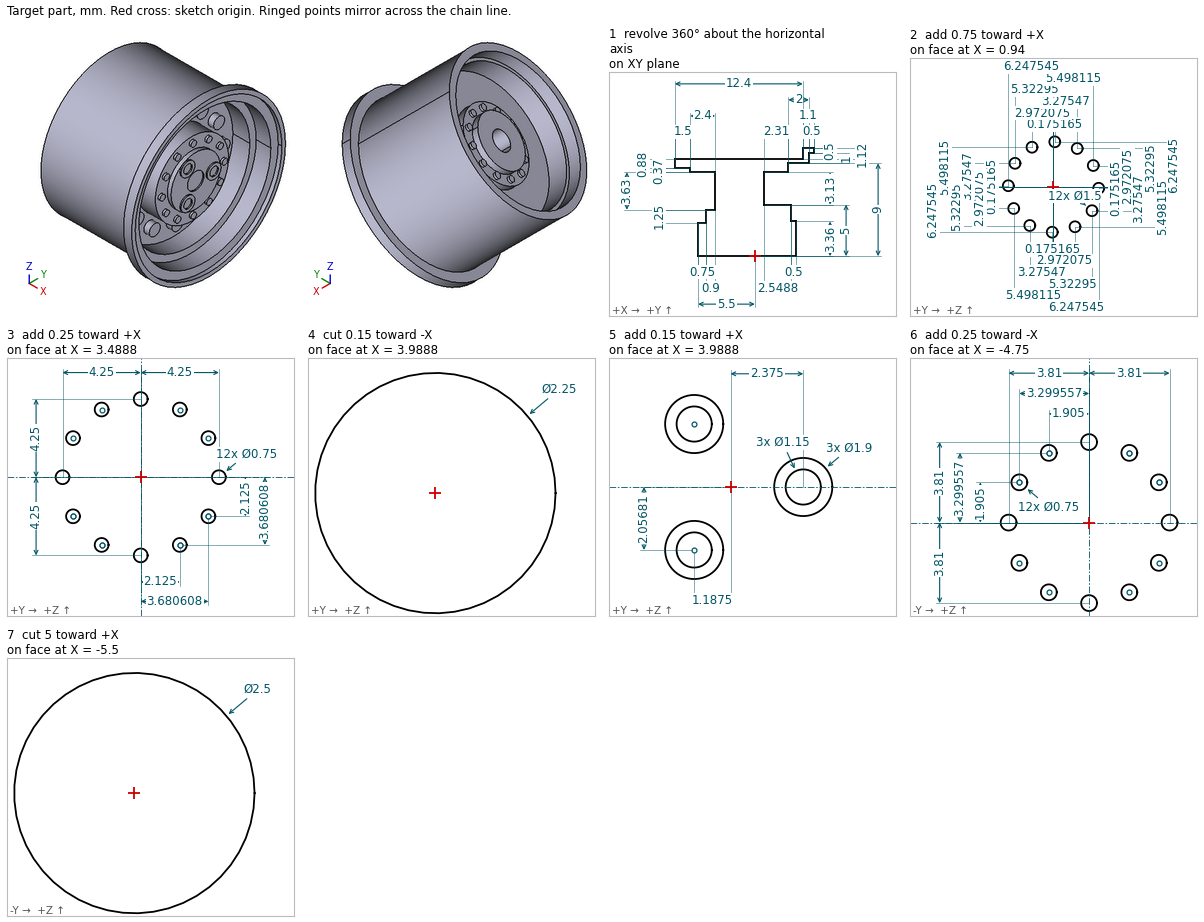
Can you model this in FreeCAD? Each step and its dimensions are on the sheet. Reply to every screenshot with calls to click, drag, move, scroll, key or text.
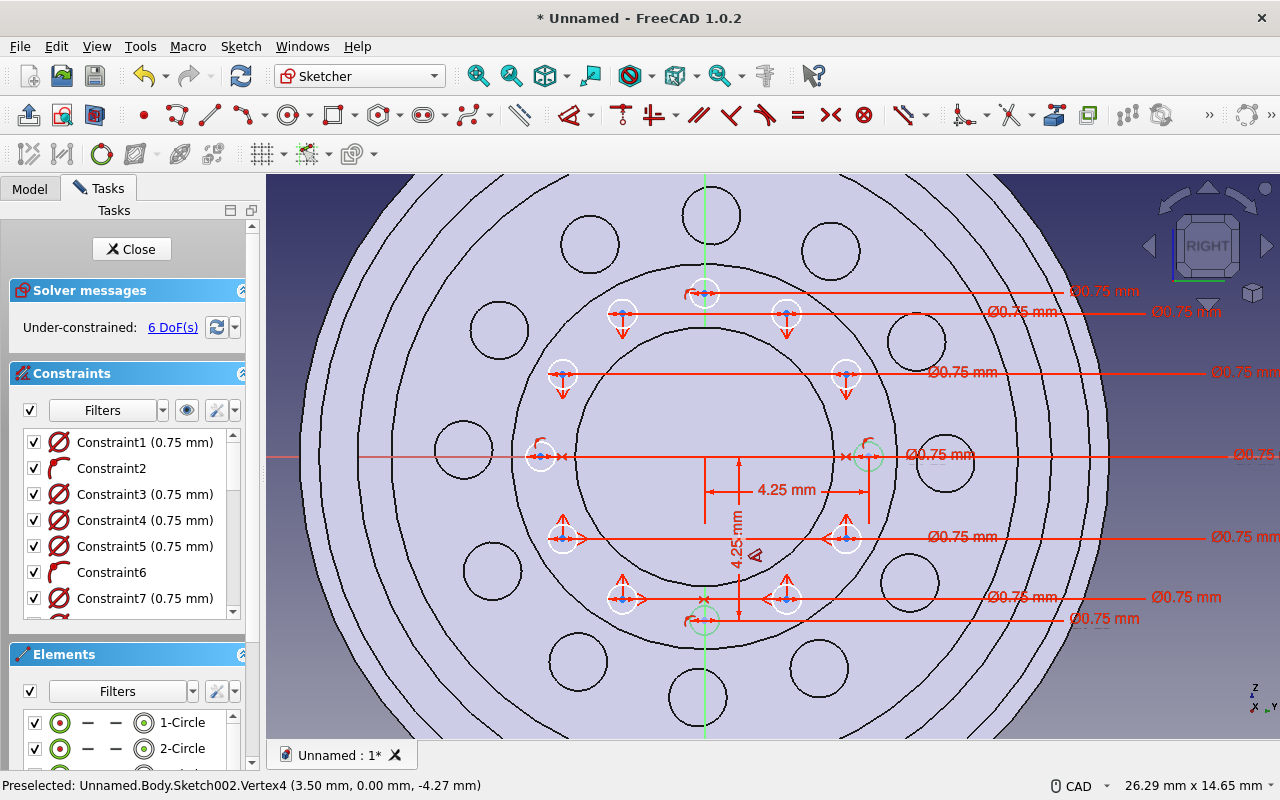
click(541, 457)
click(623, 491)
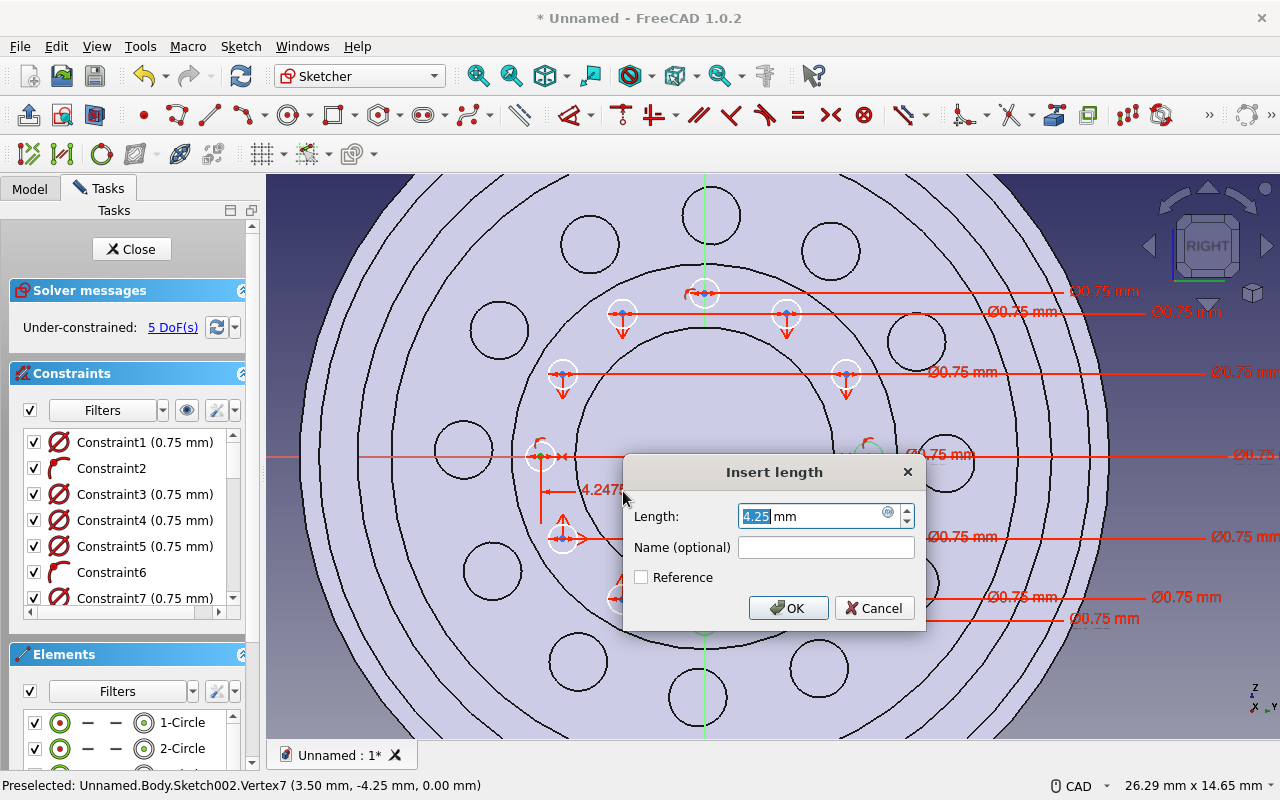
text(4.25)
key(Return)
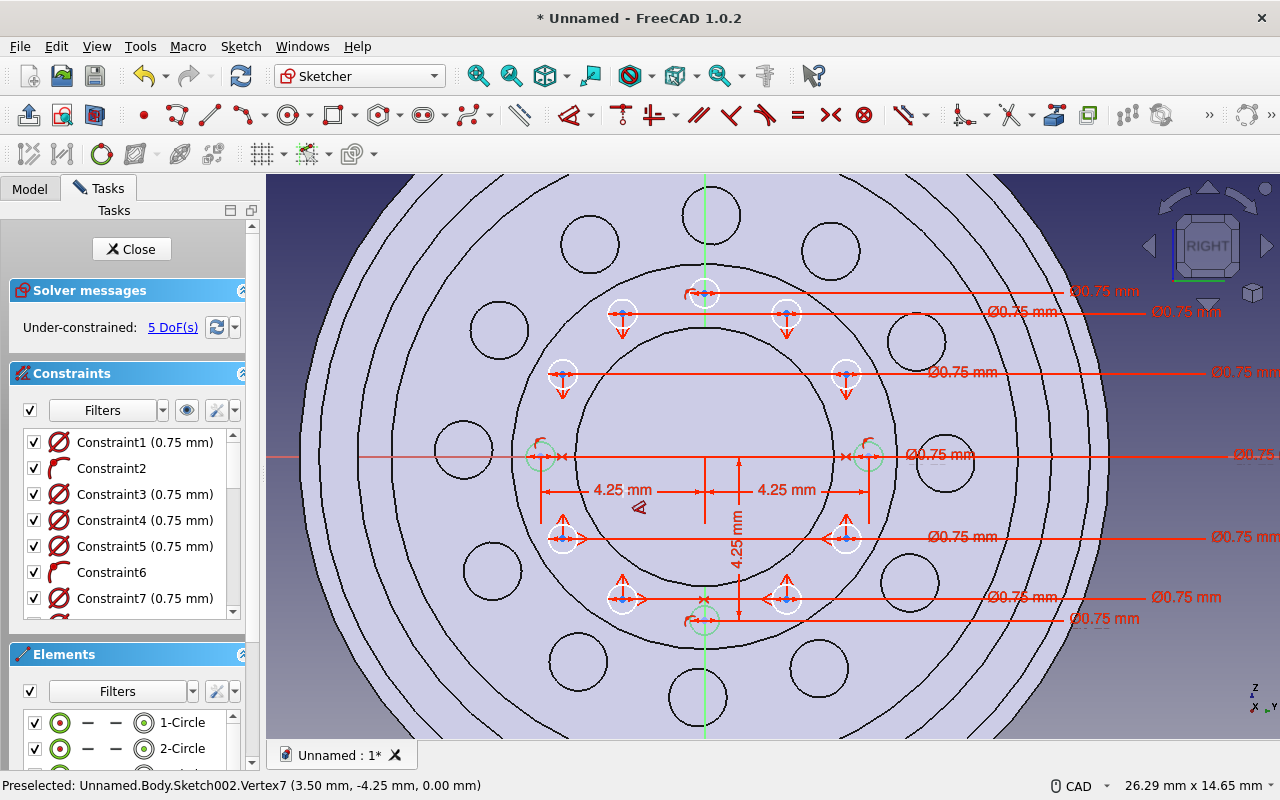
click(705, 293)
click(739, 375)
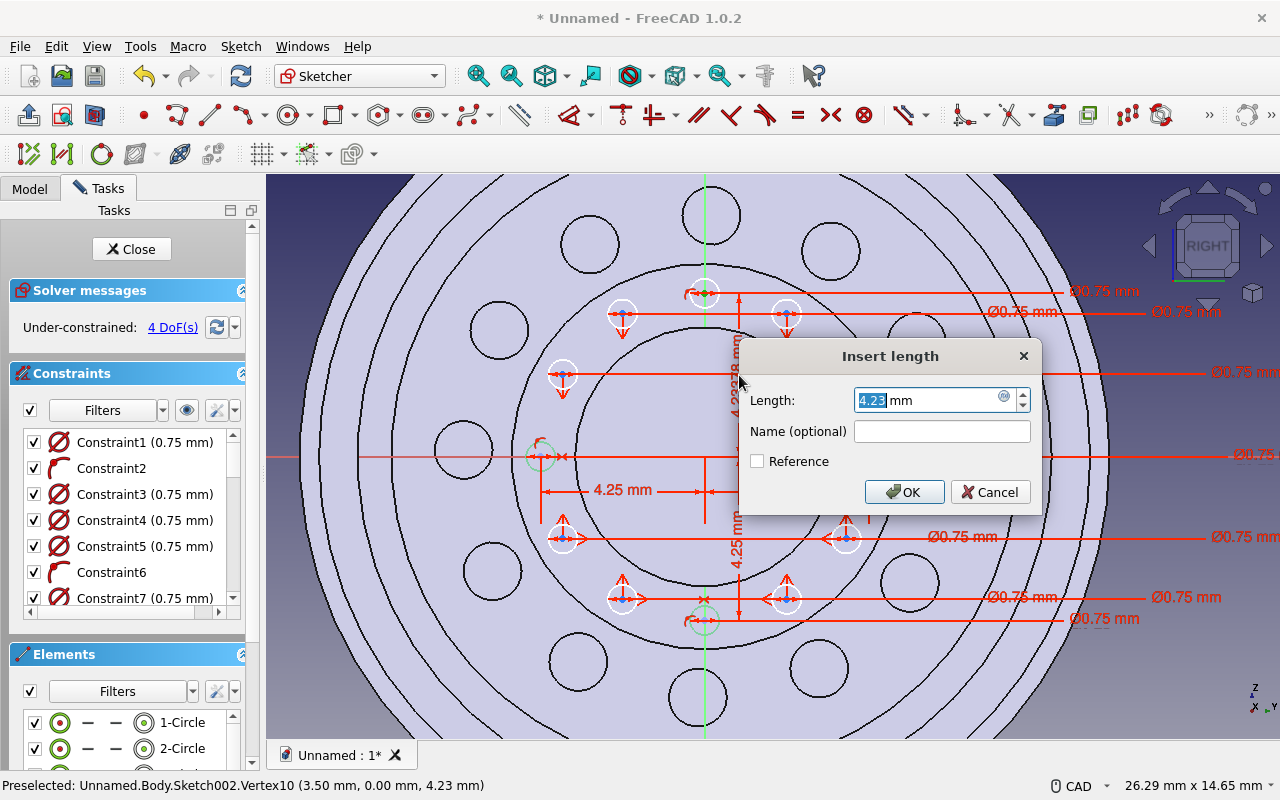
text(4.25)
key(Return)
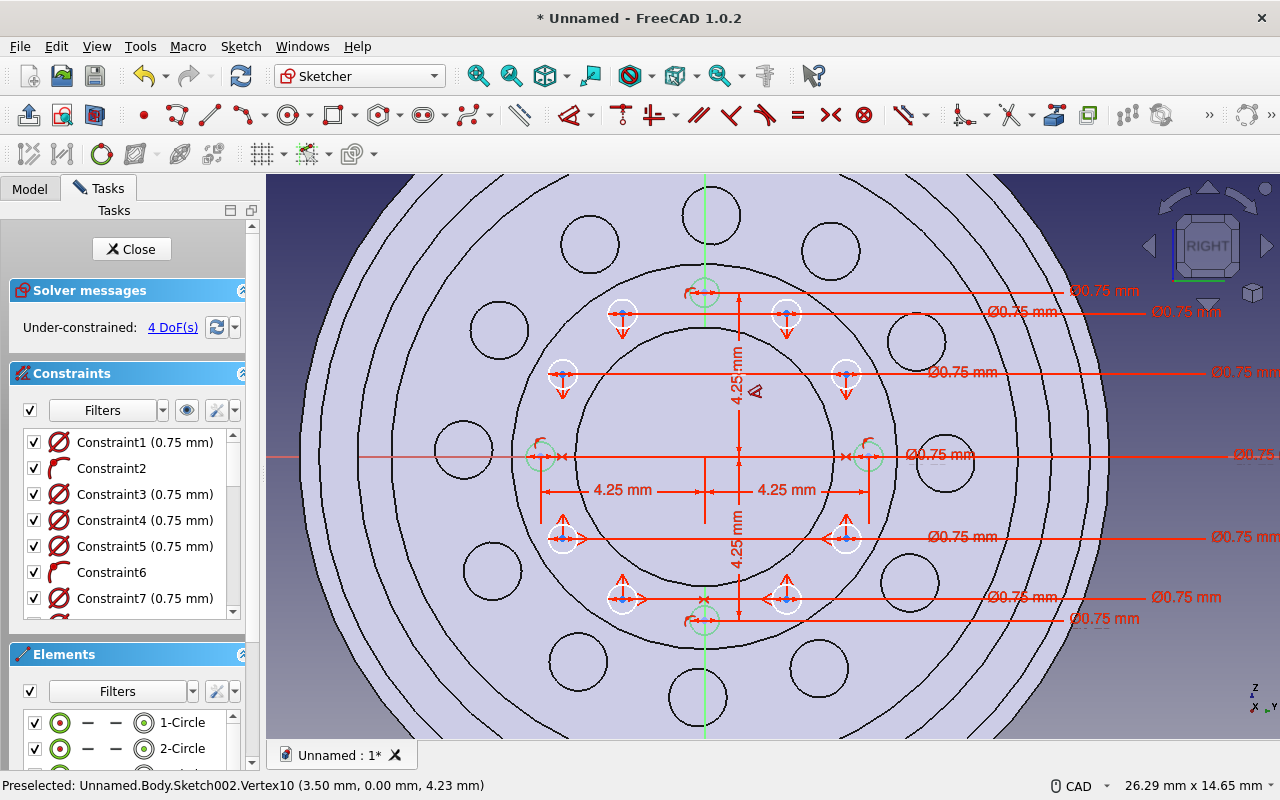
click(846, 539)
click(880, 498)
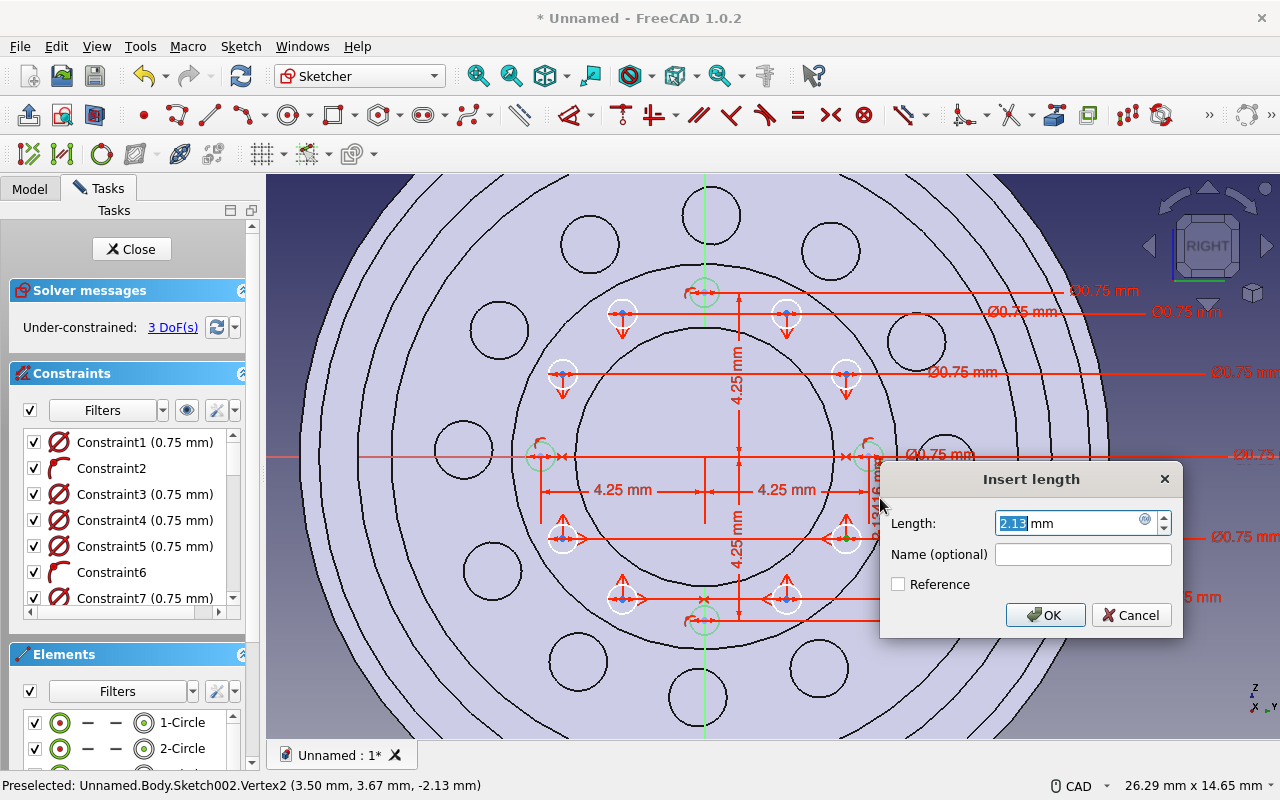
text(2.125)
key(Return)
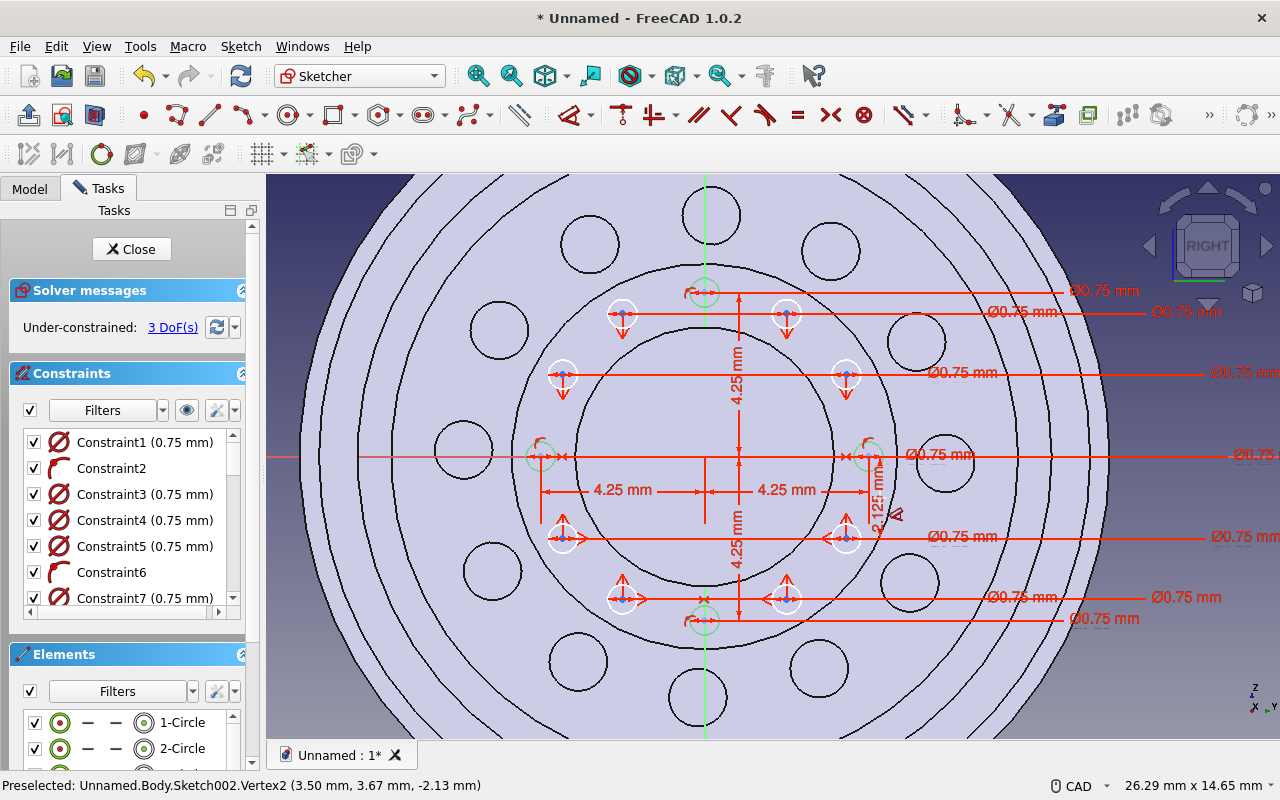
click(787, 599)
click(746, 633)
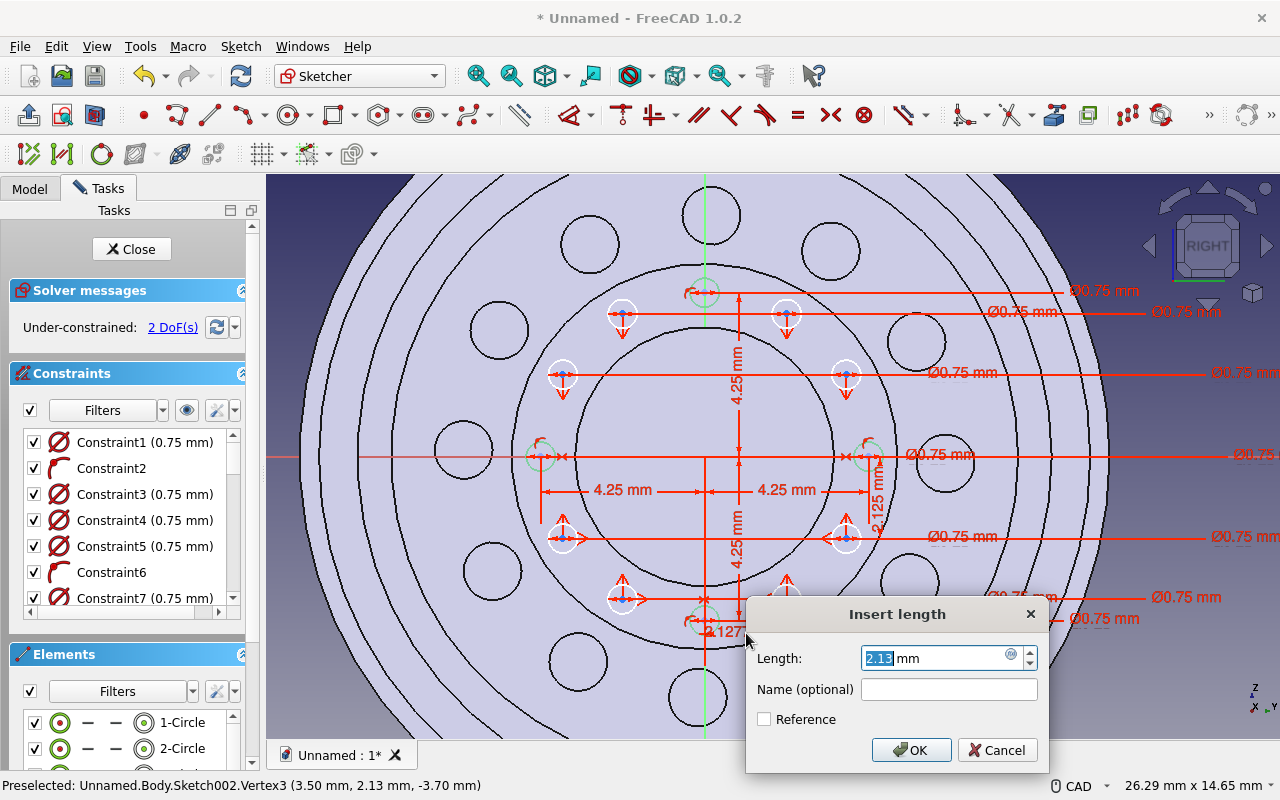
text(2.125)
key(Return)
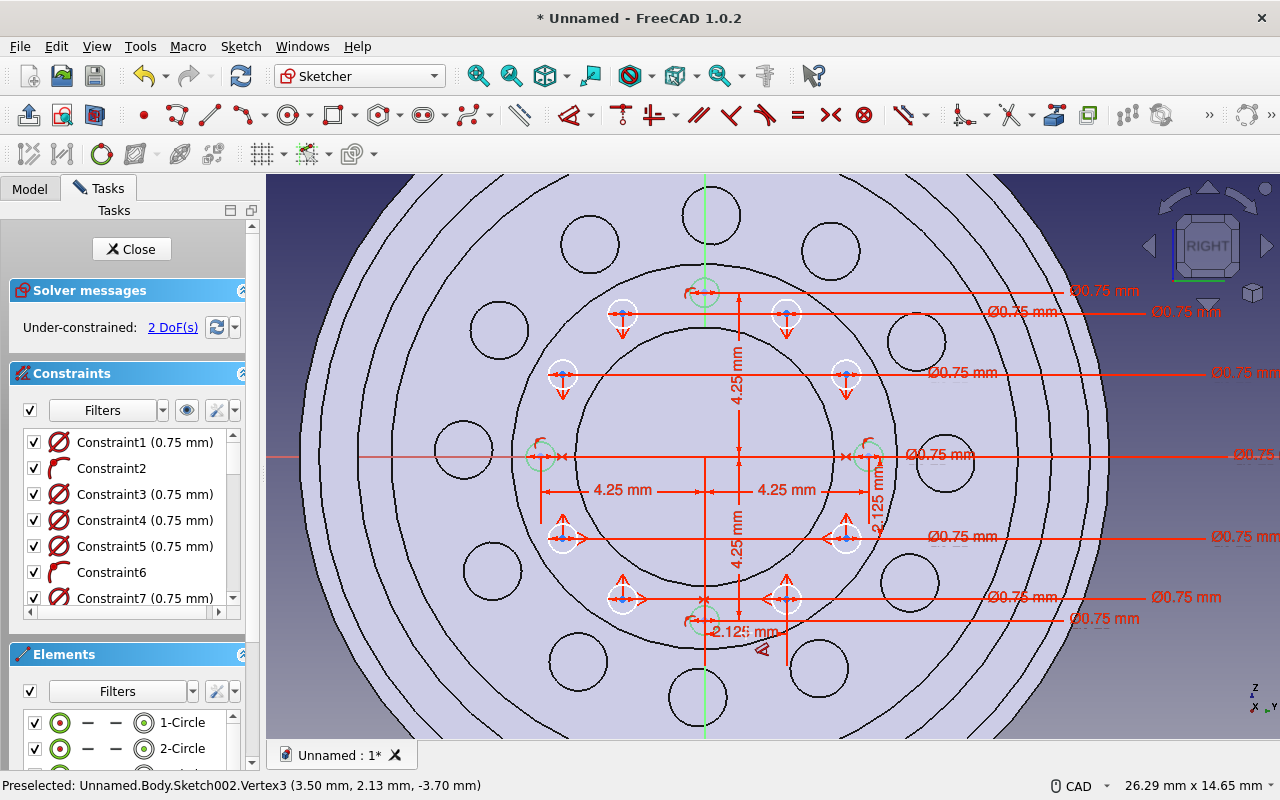
click(846, 539)
click(775, 573)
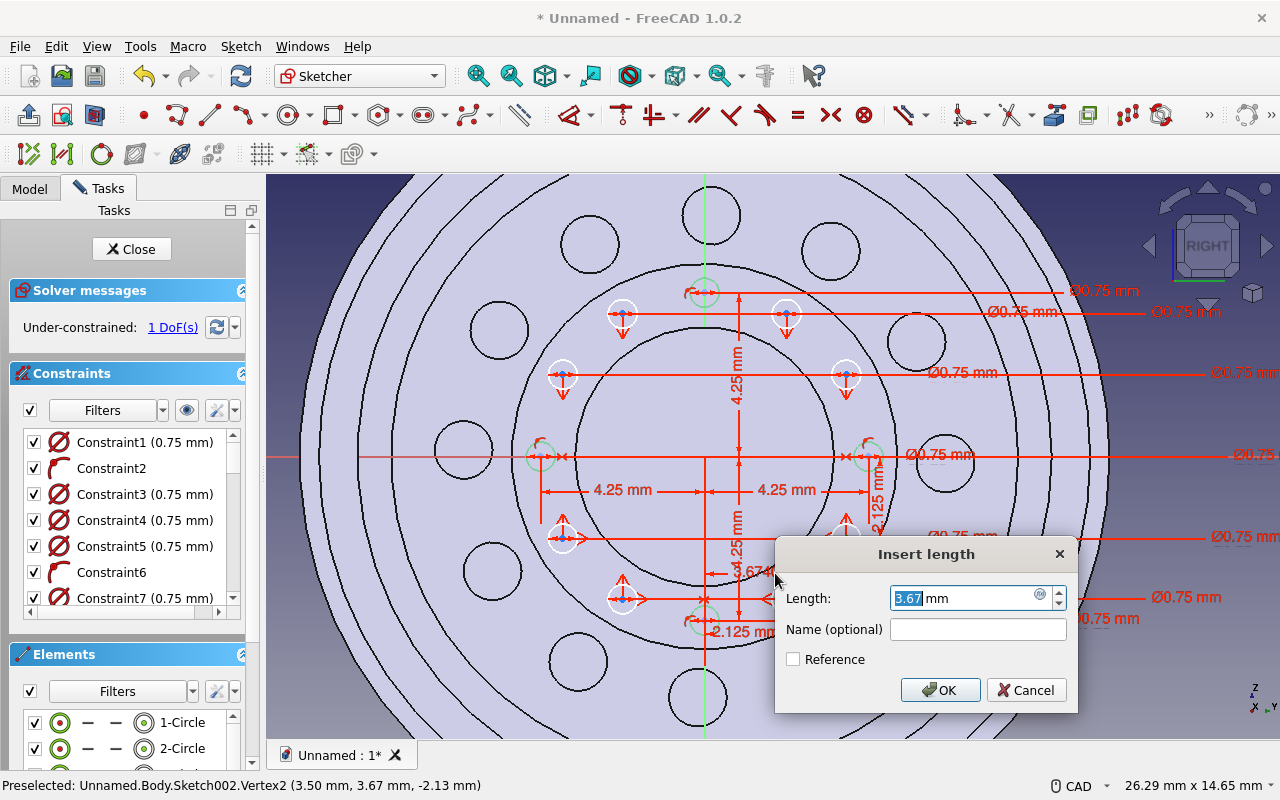
text(3.680608)
key(Return)